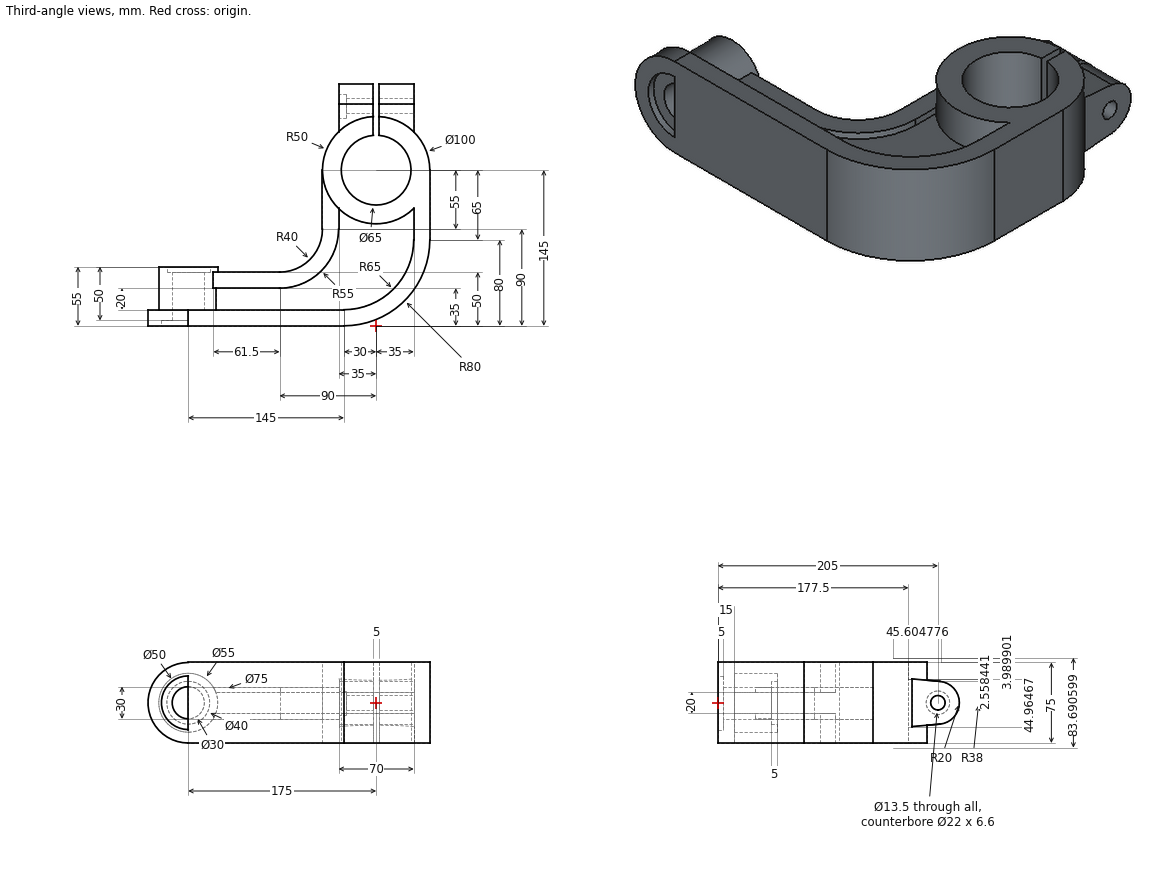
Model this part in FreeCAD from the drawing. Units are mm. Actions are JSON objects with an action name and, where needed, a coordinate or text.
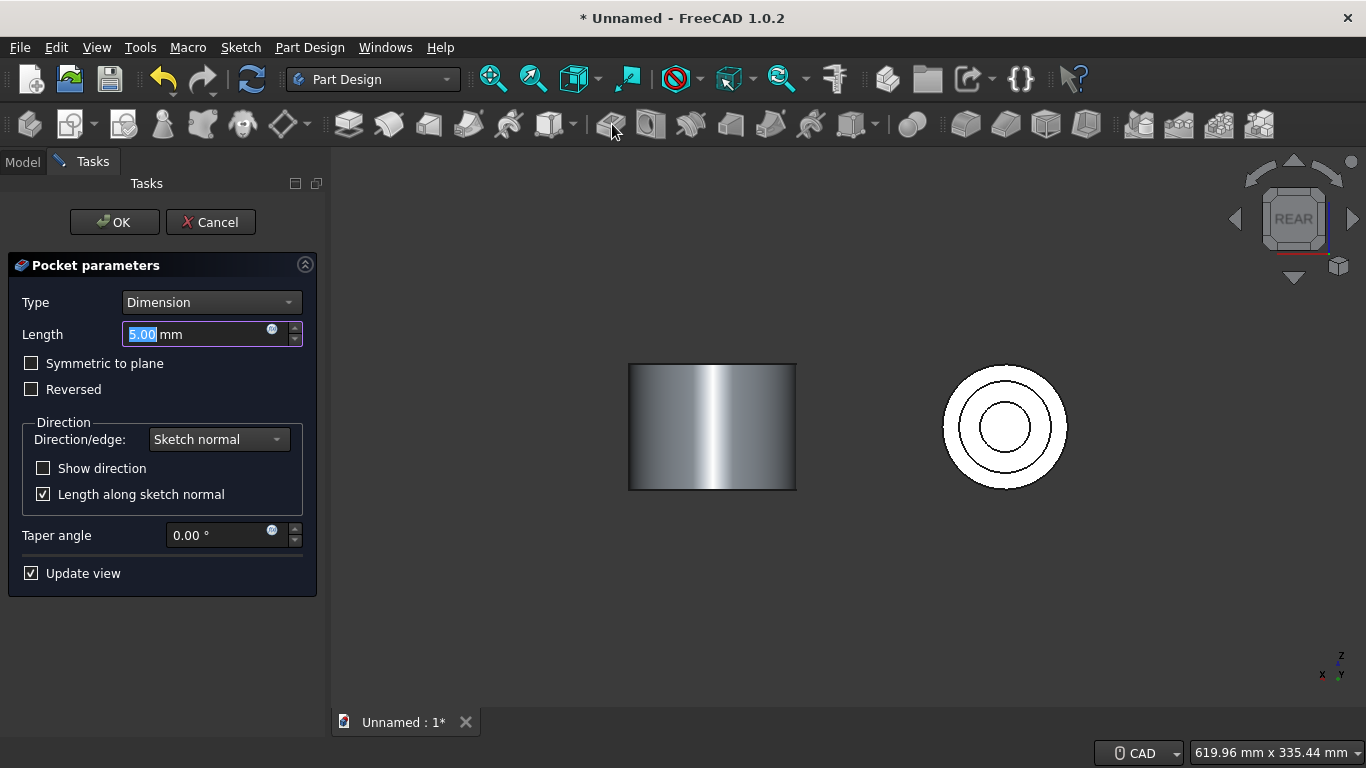
{"action": "type", "text": "50"}
{"action": "key", "text": "Tab"}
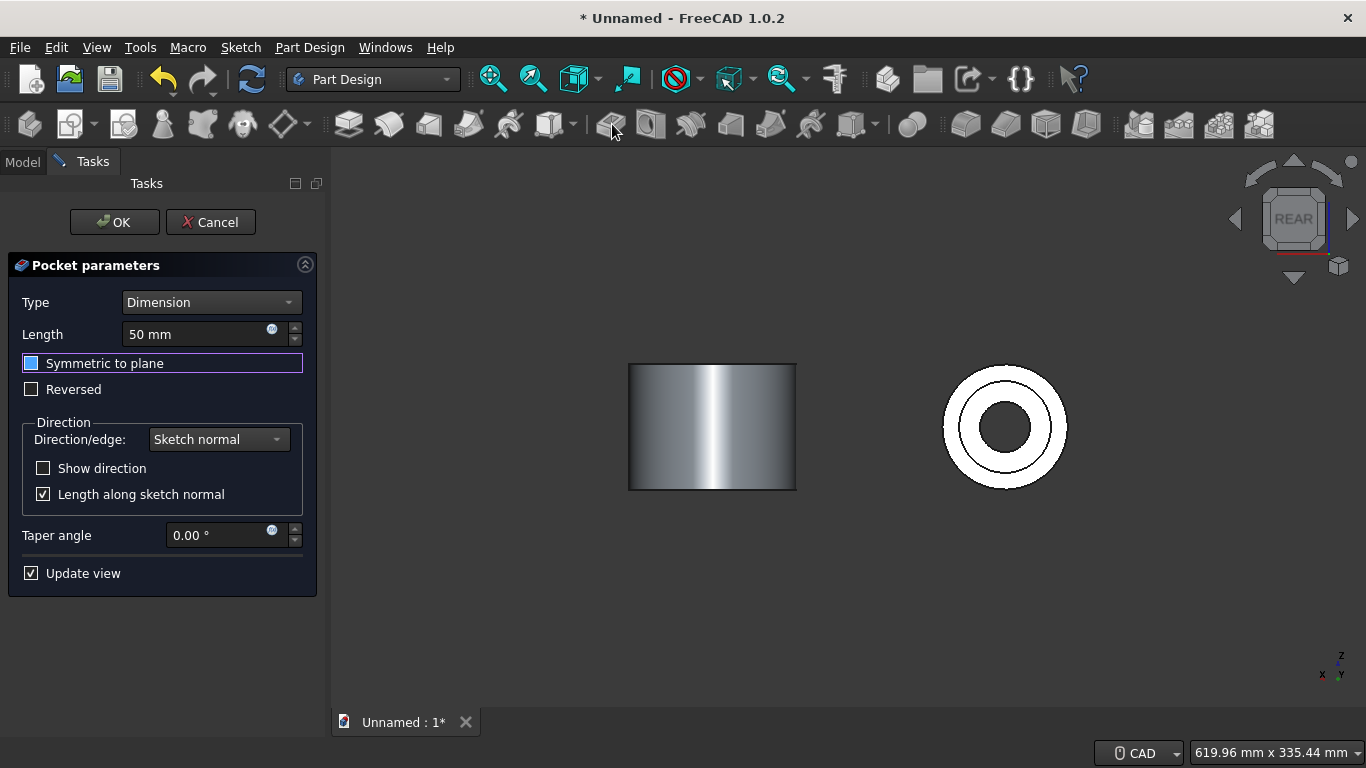
{"action": "left_click", "coordinate": [115, 222]}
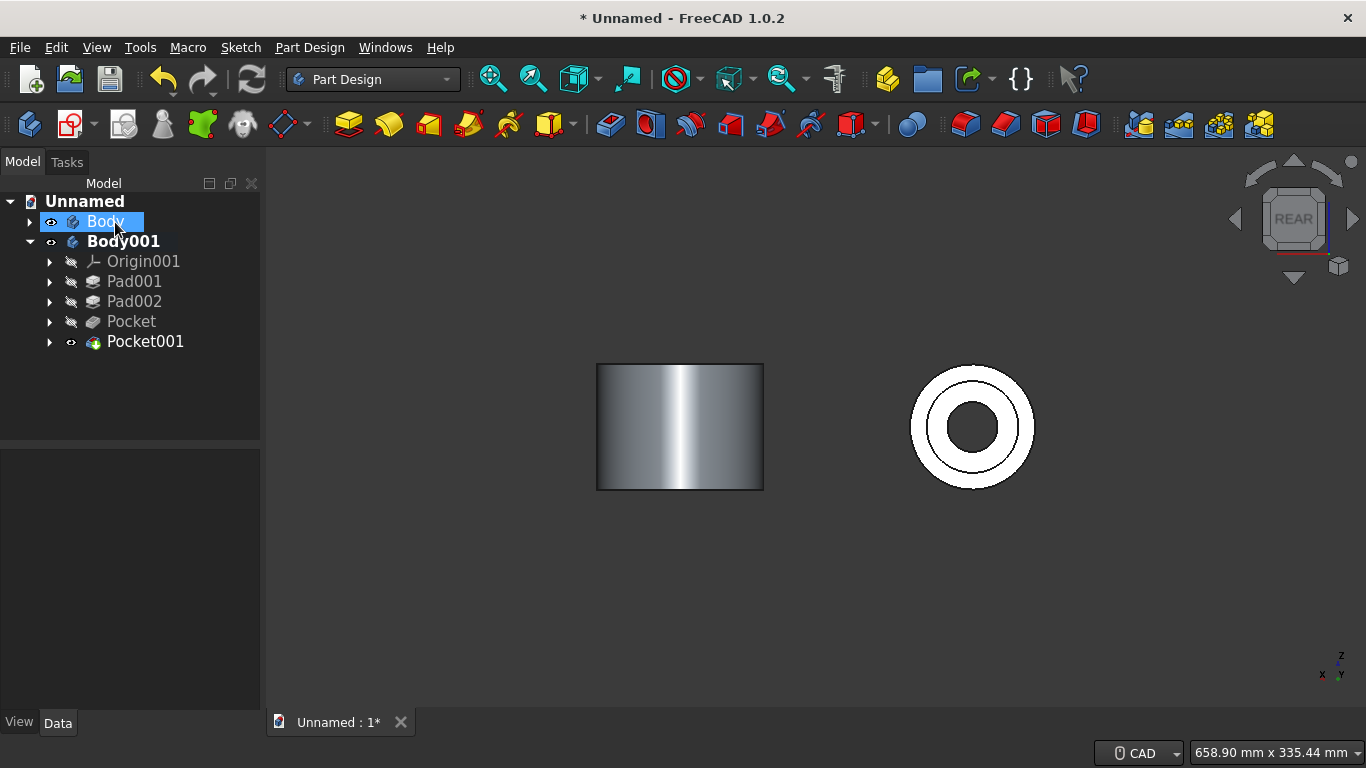
{"action": "key", "text": "v f"}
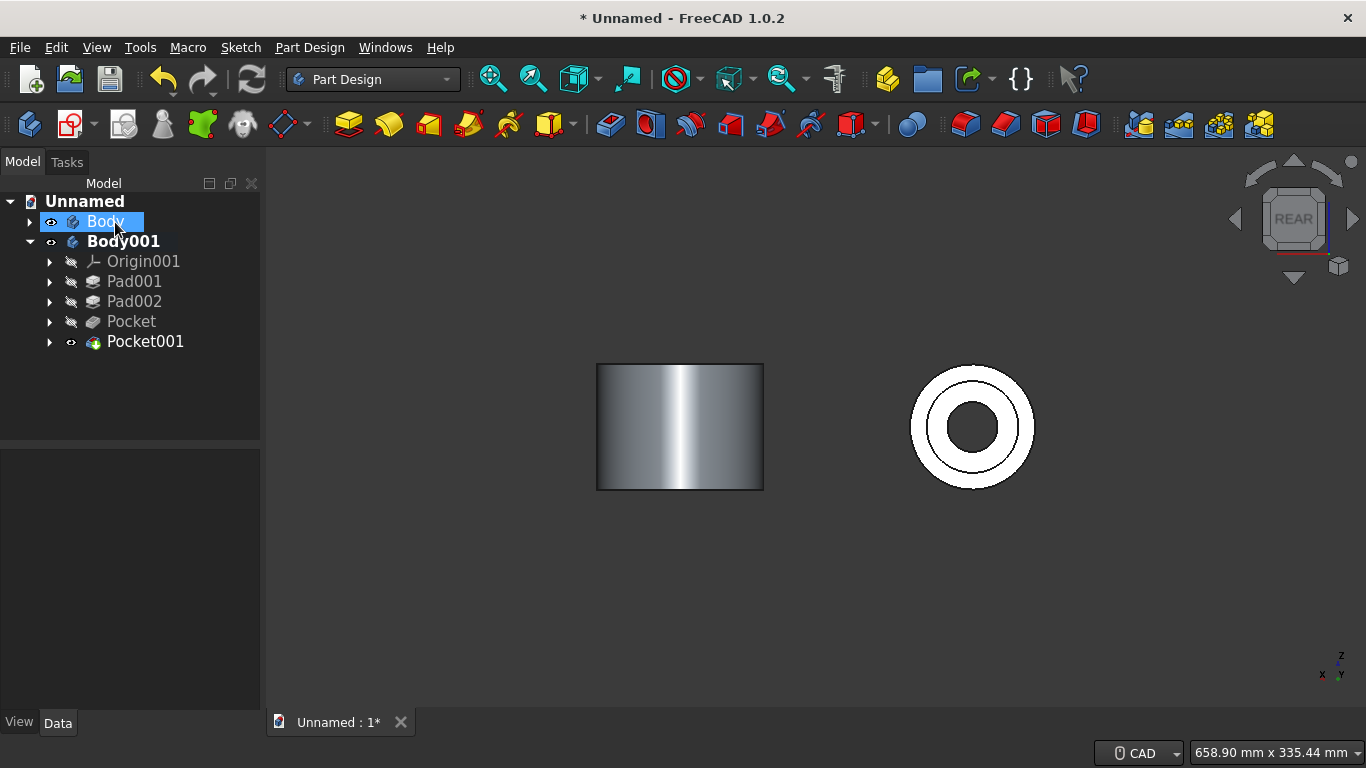
{"action": "left_click", "coordinate": [946, 400]}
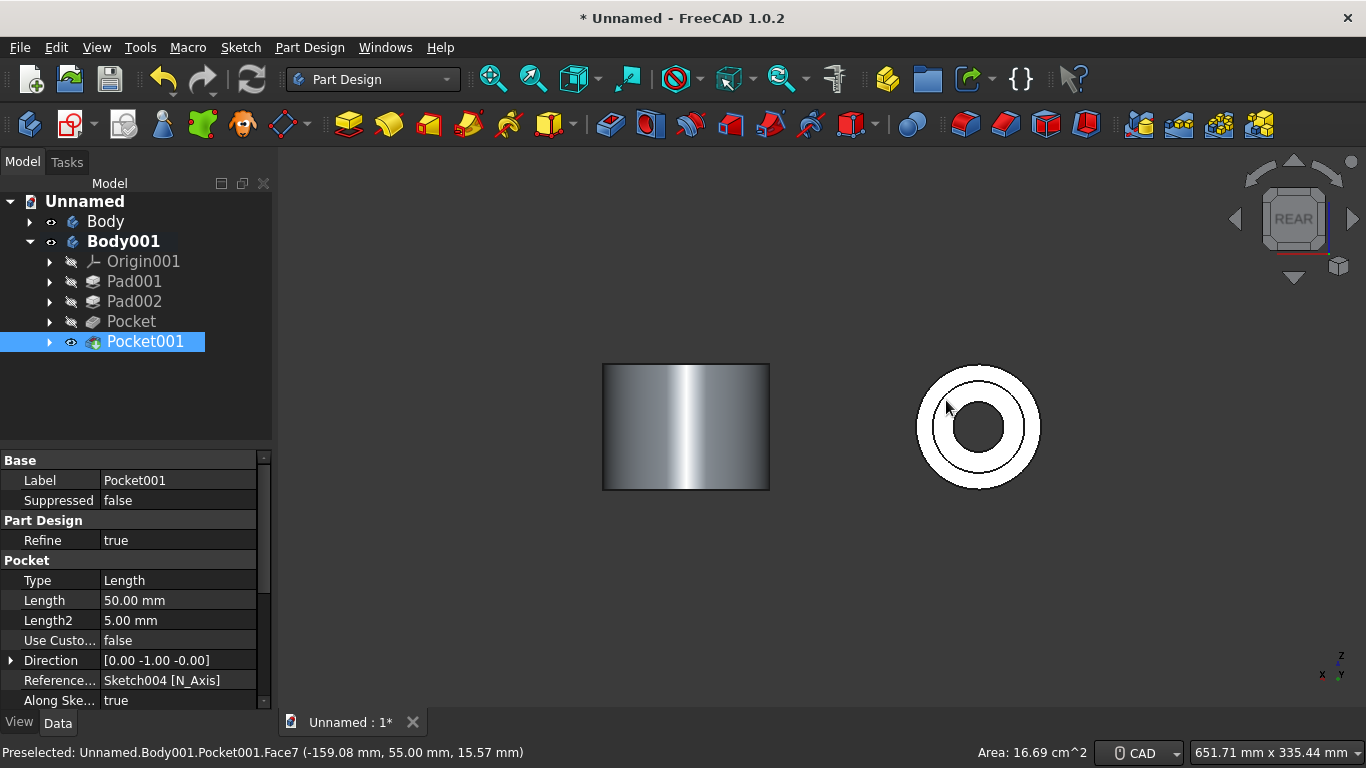
{"action": "left_click", "coordinate": [70, 124]}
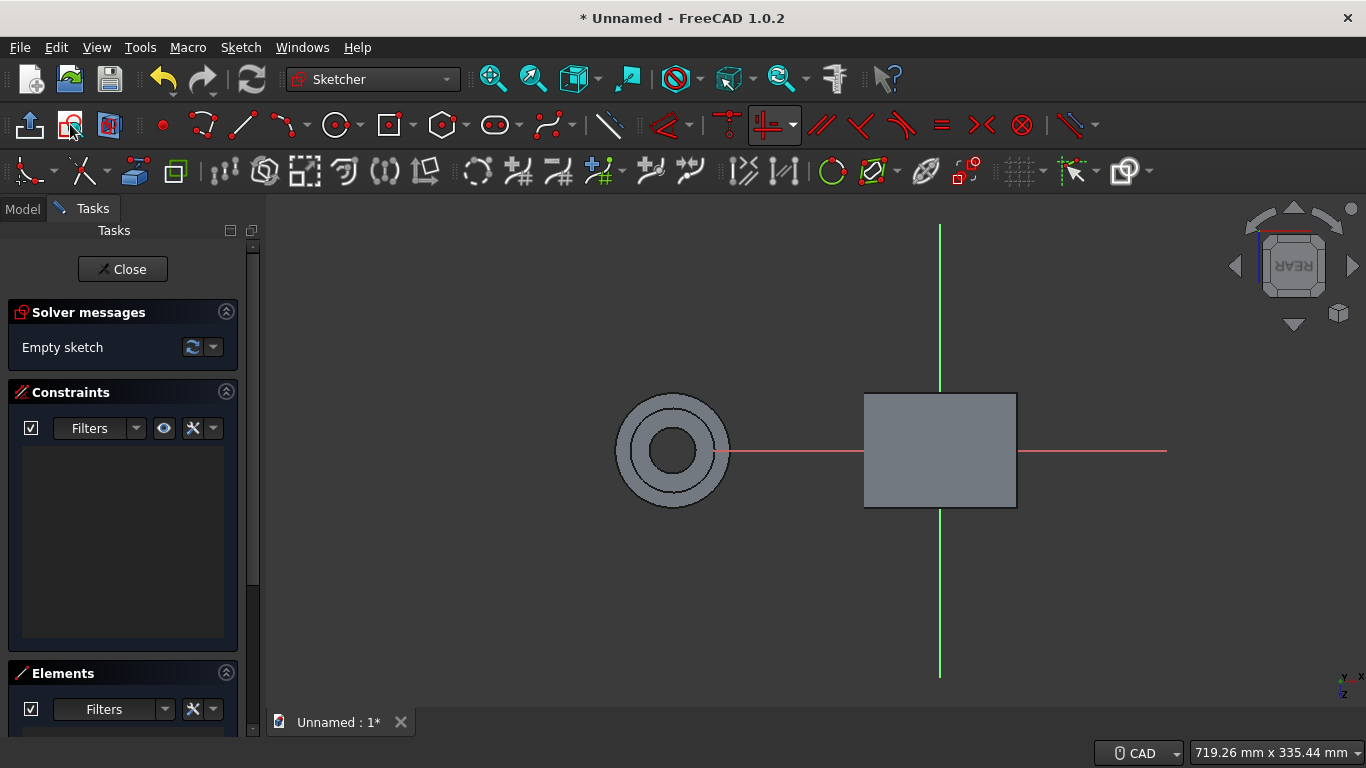
{"action": "scroll", "coordinate": [654, 450], "scroll_direction": "up", "scroll_amount": 8}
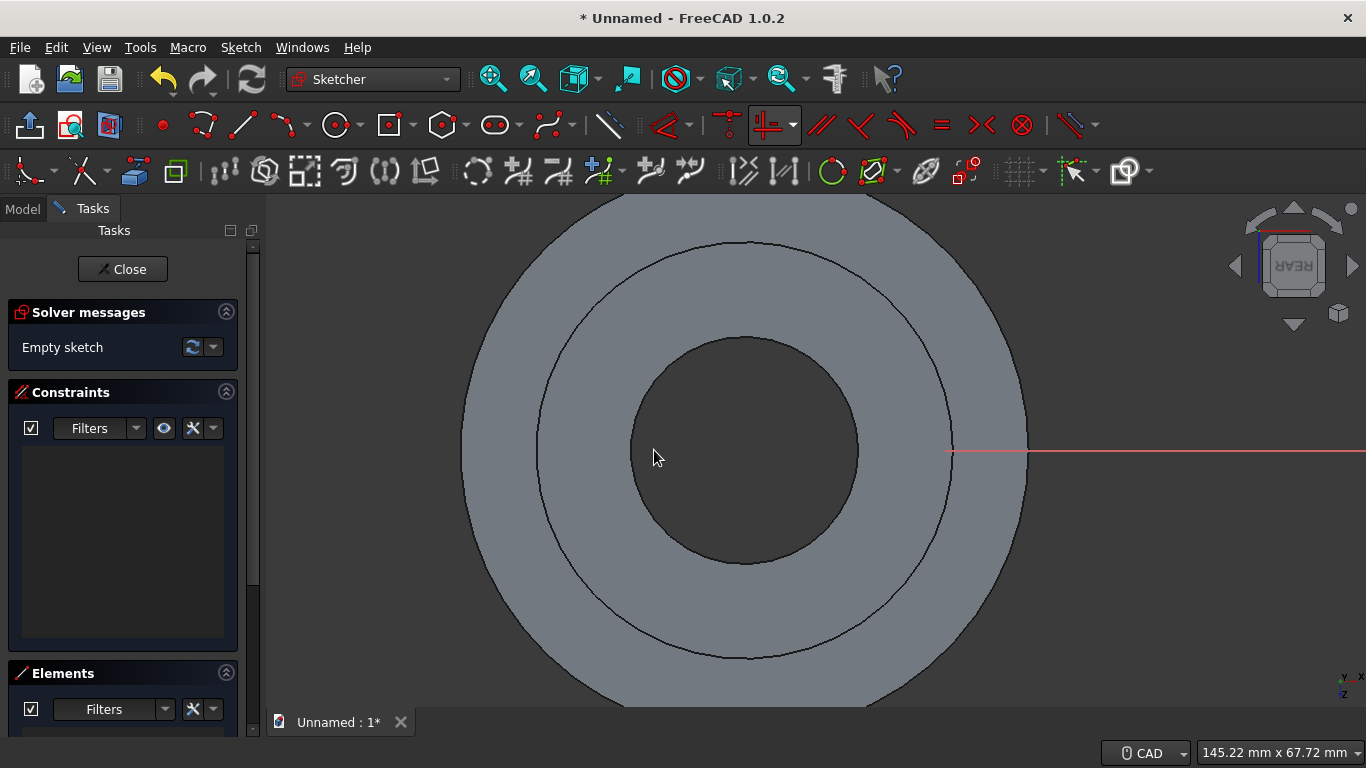
{"action": "left_click", "coordinate": [336, 126]}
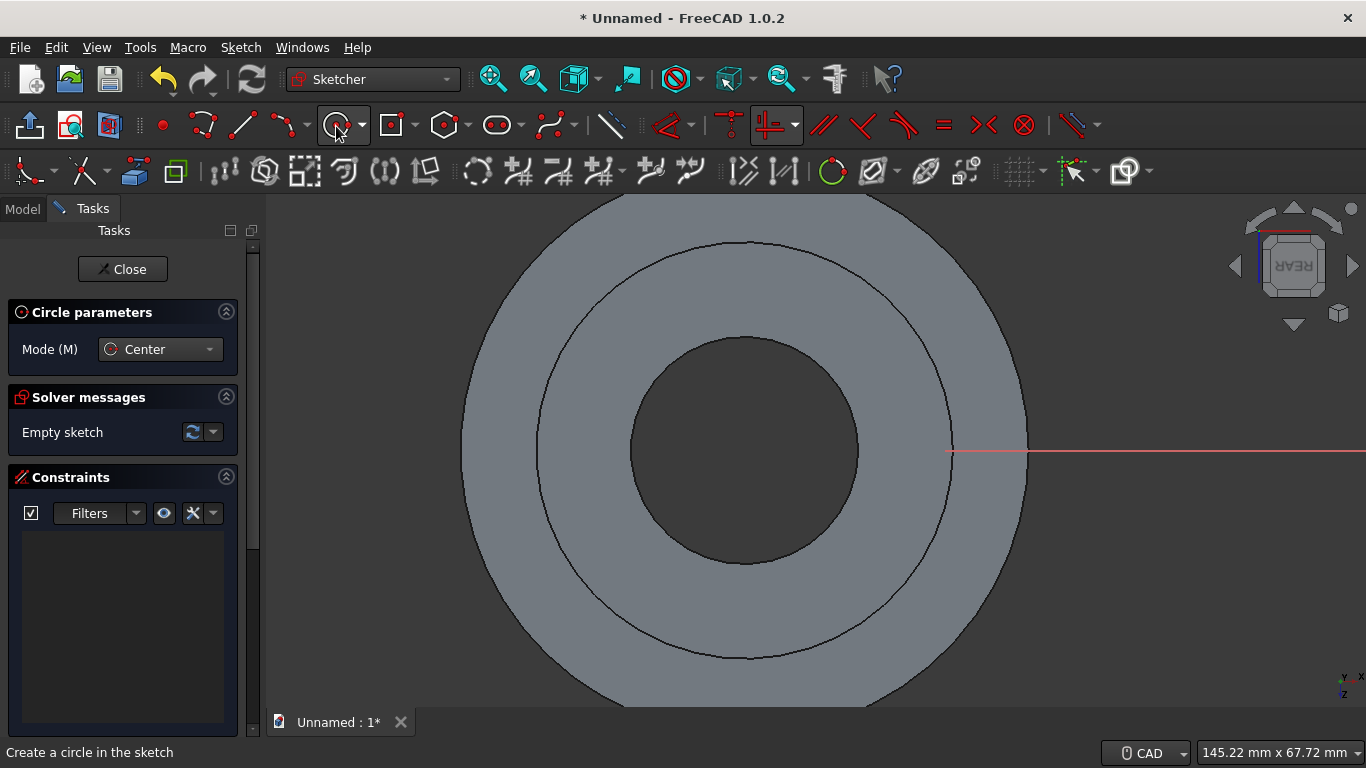
{"action": "left_click", "coordinate": [745, 450]}
{"action": "left_click", "coordinate": [852, 343]}
{"action": "key", "text": "Escape"}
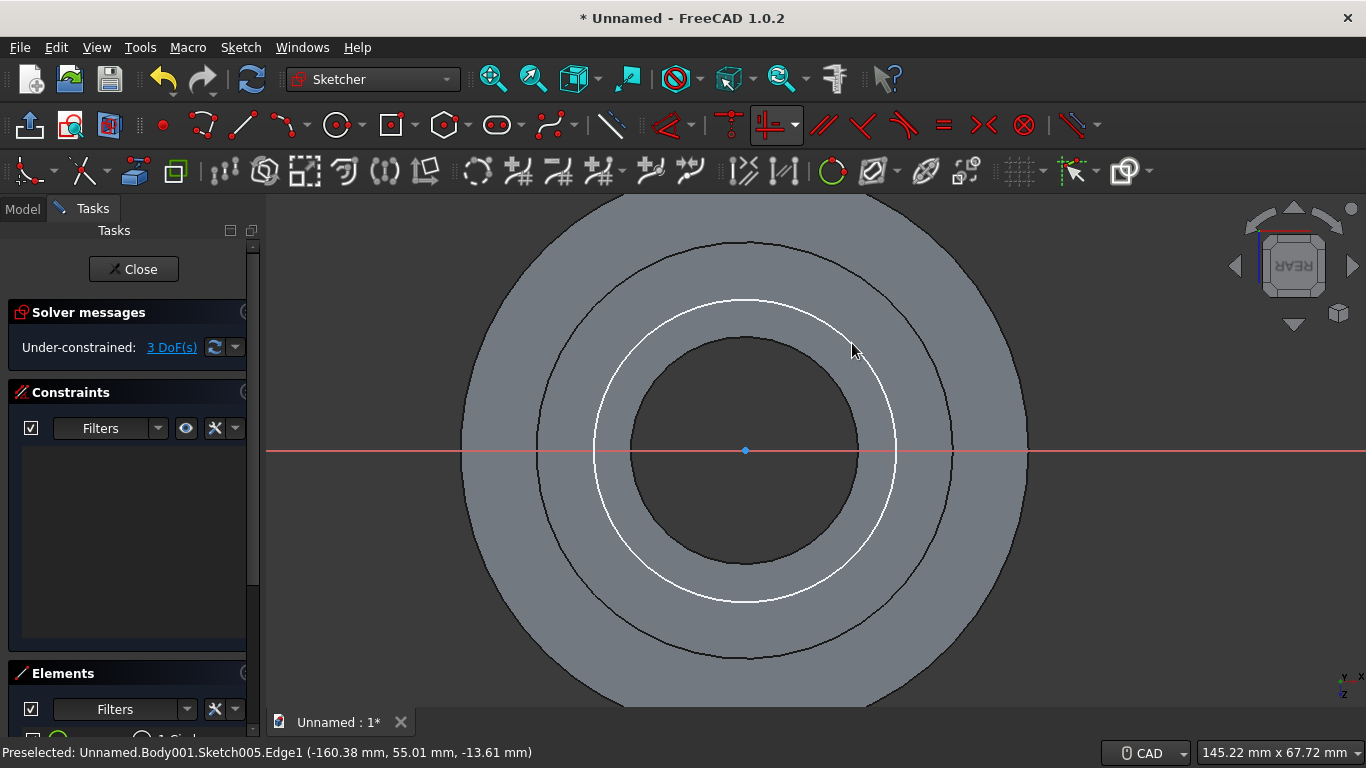
{"action": "left_click", "coordinate": [745, 451]}